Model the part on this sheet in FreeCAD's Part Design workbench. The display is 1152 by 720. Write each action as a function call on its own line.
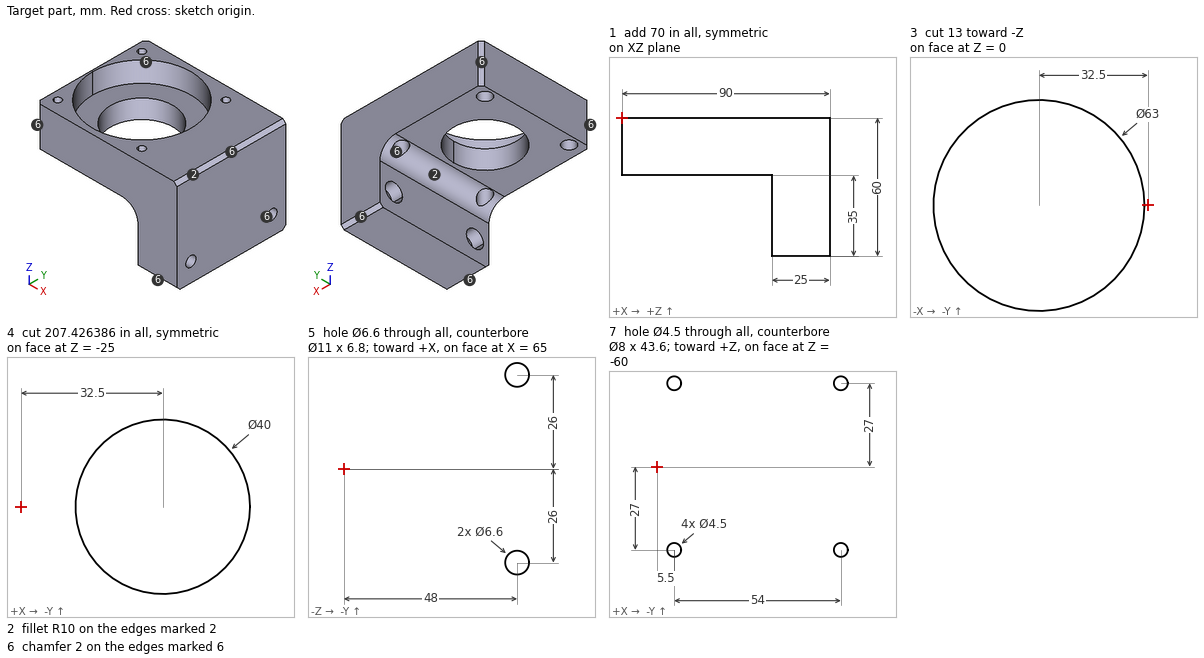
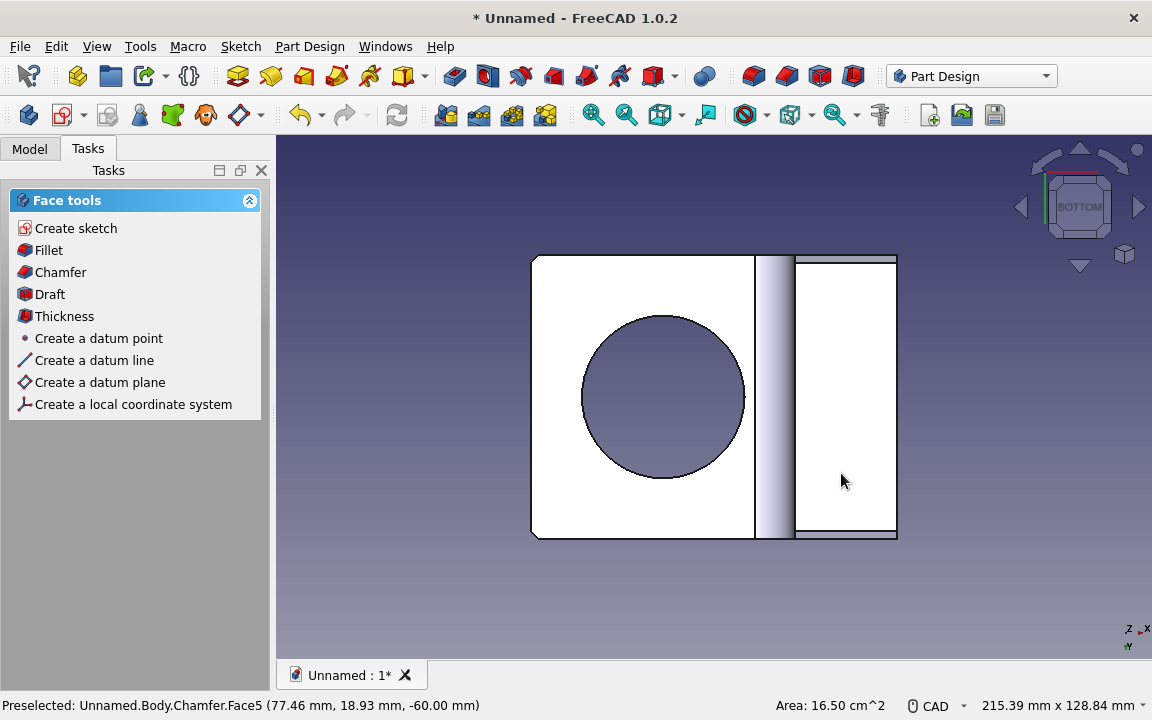
click(62, 116)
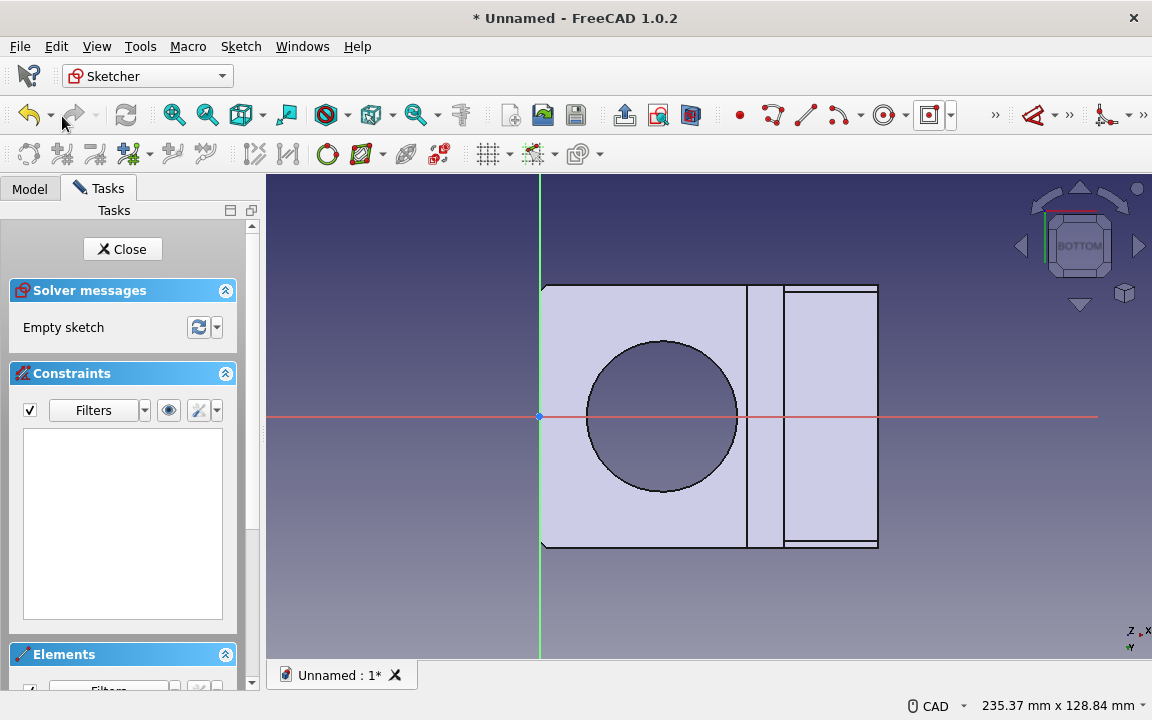
scroll(687, 417, up, 2)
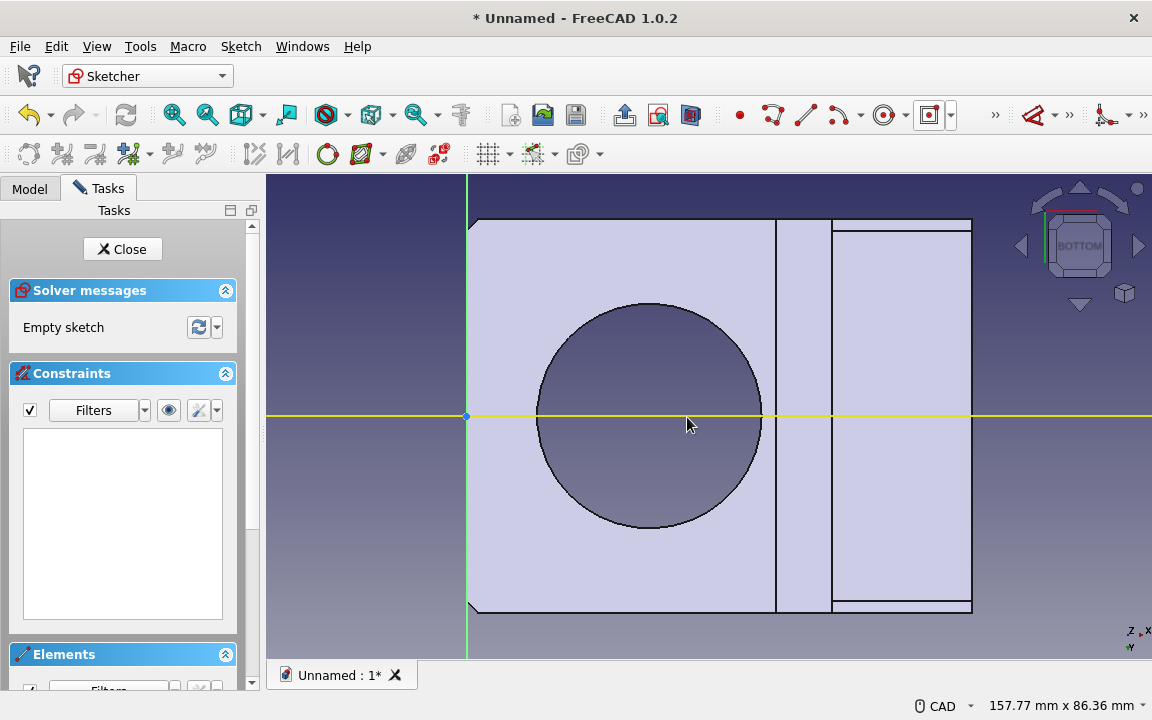
click(884, 116)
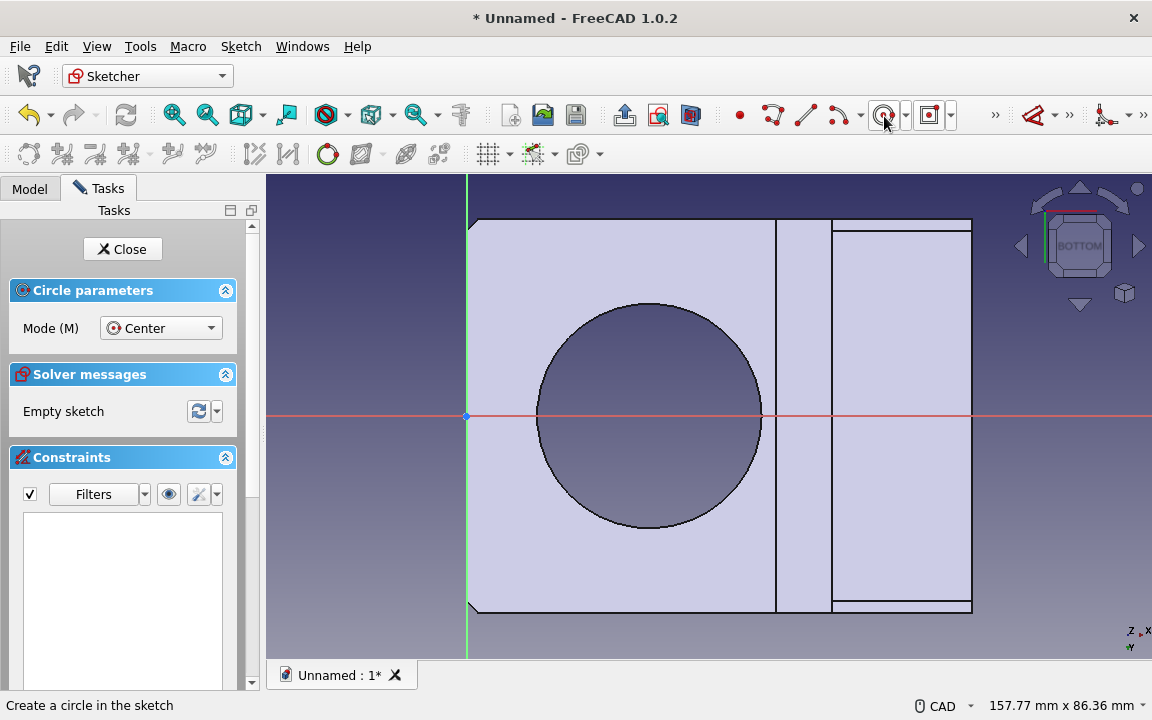
scroll(498, 568, up, 3)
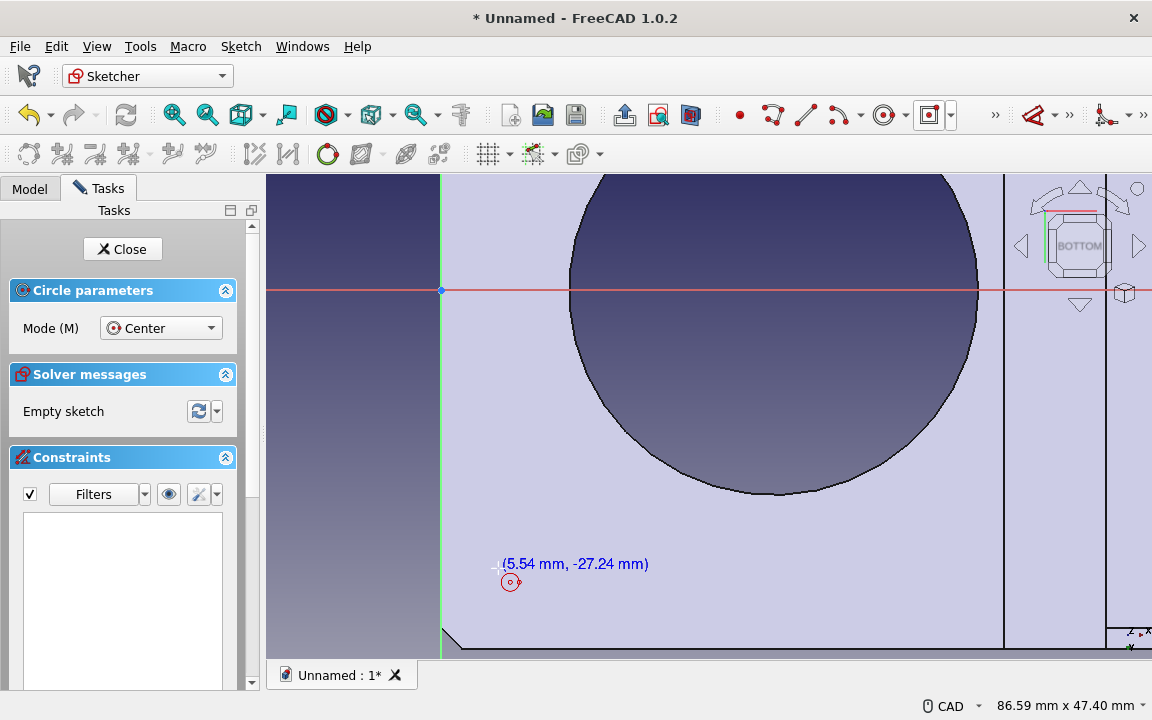
click(497, 567)
move(514, 550)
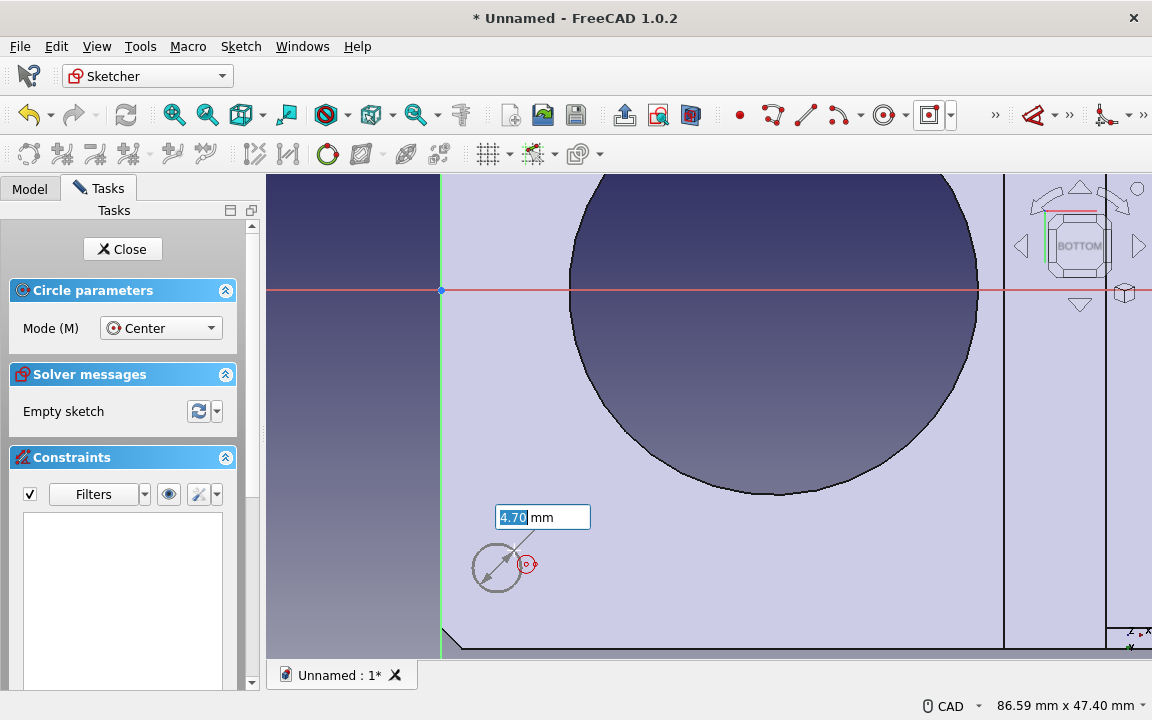
text(4.5)
key(Return)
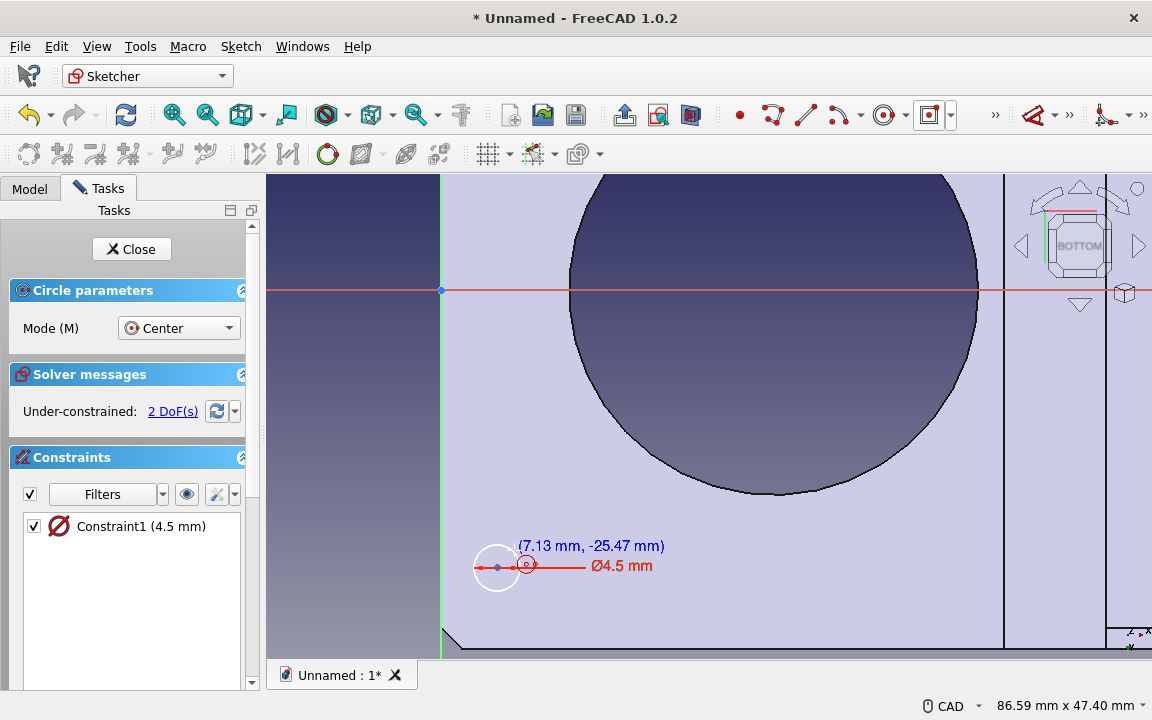
scroll(499, 570, down, 3)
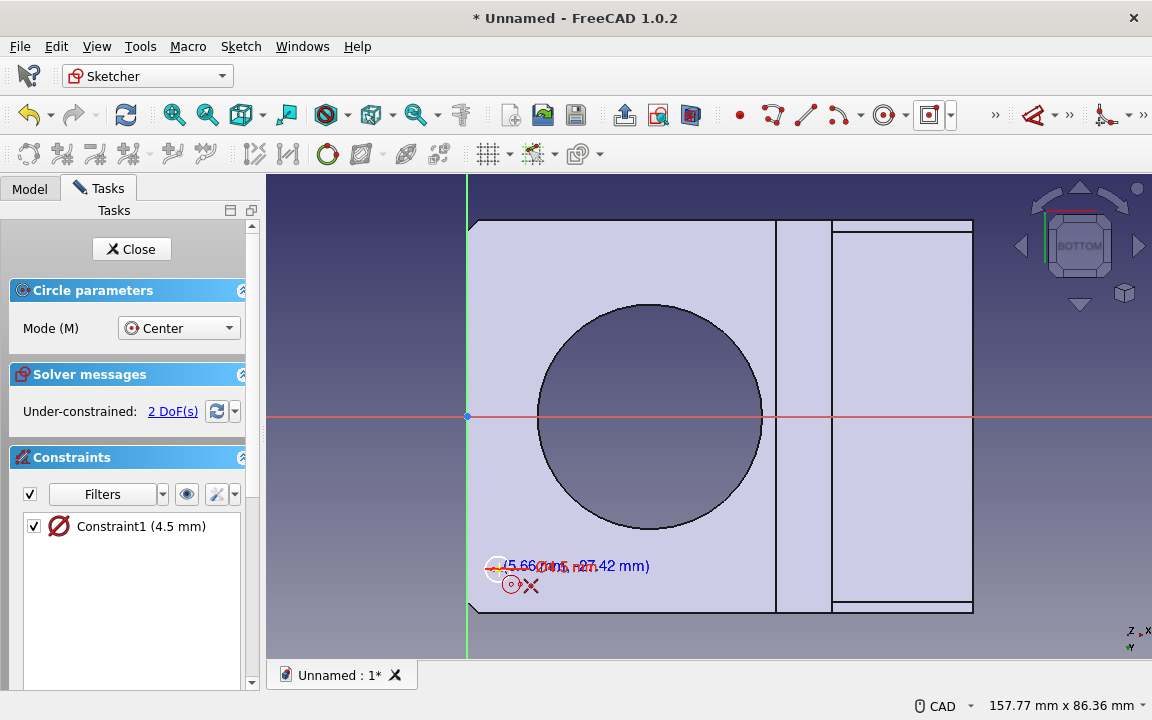
scroll(801, 569, up, 3)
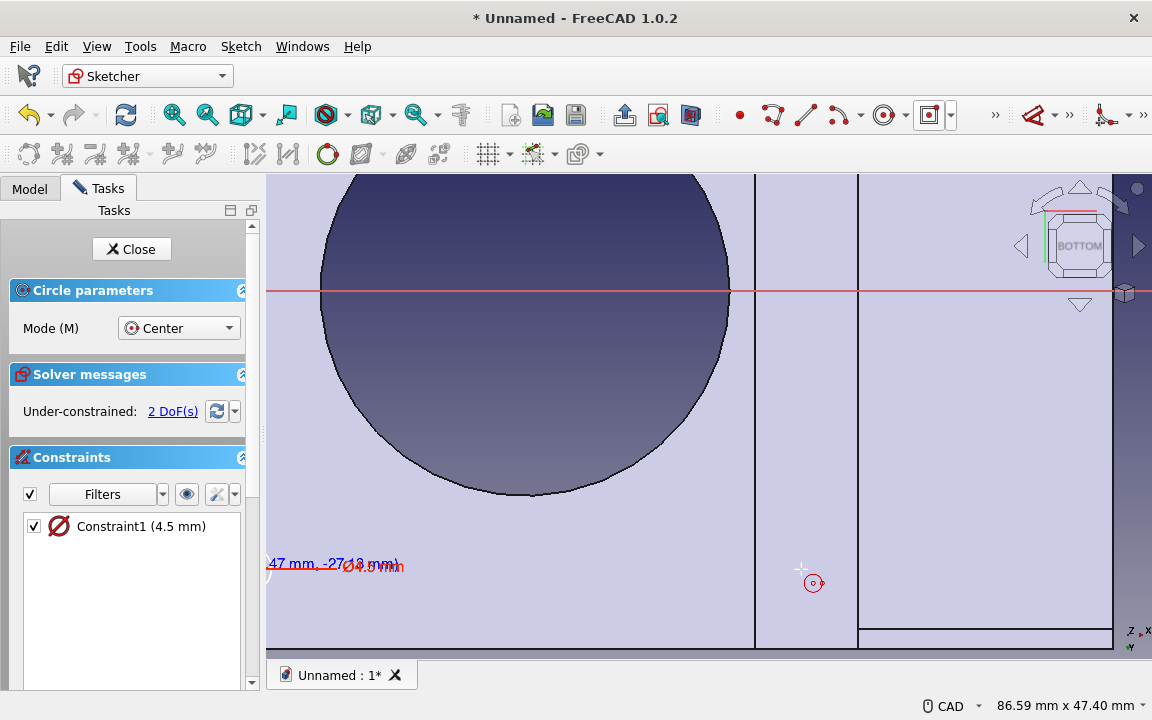
click(801, 567)
move(818, 551)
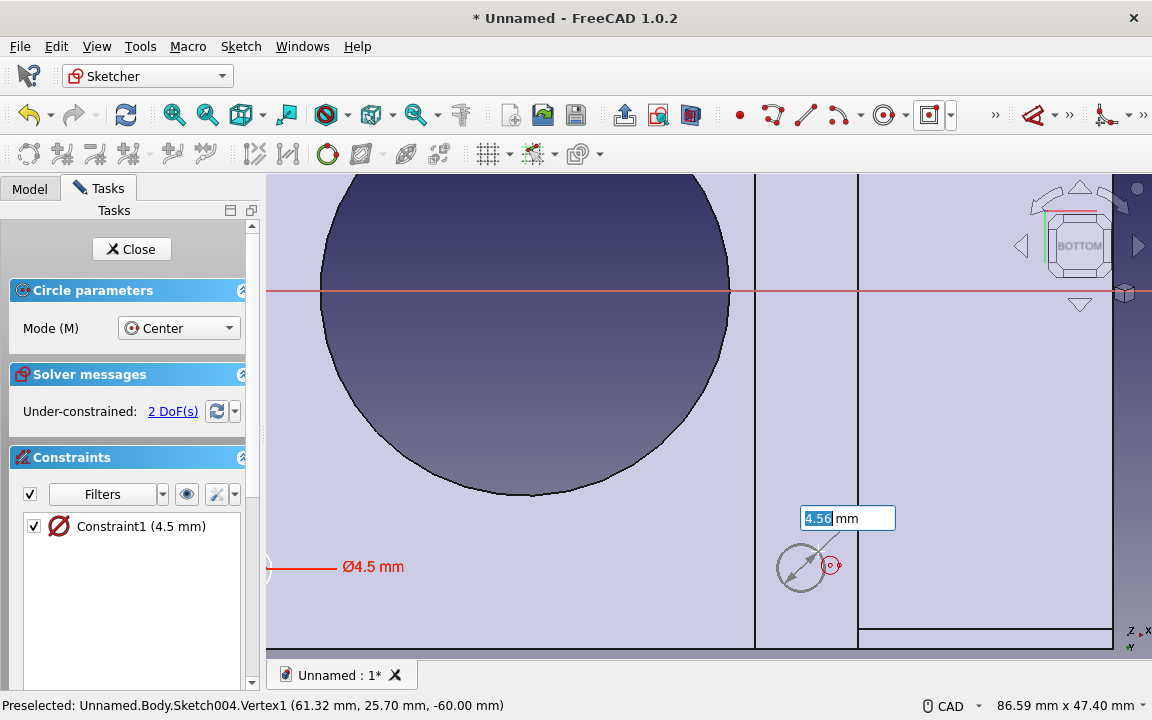
text(4.5)
key(Return)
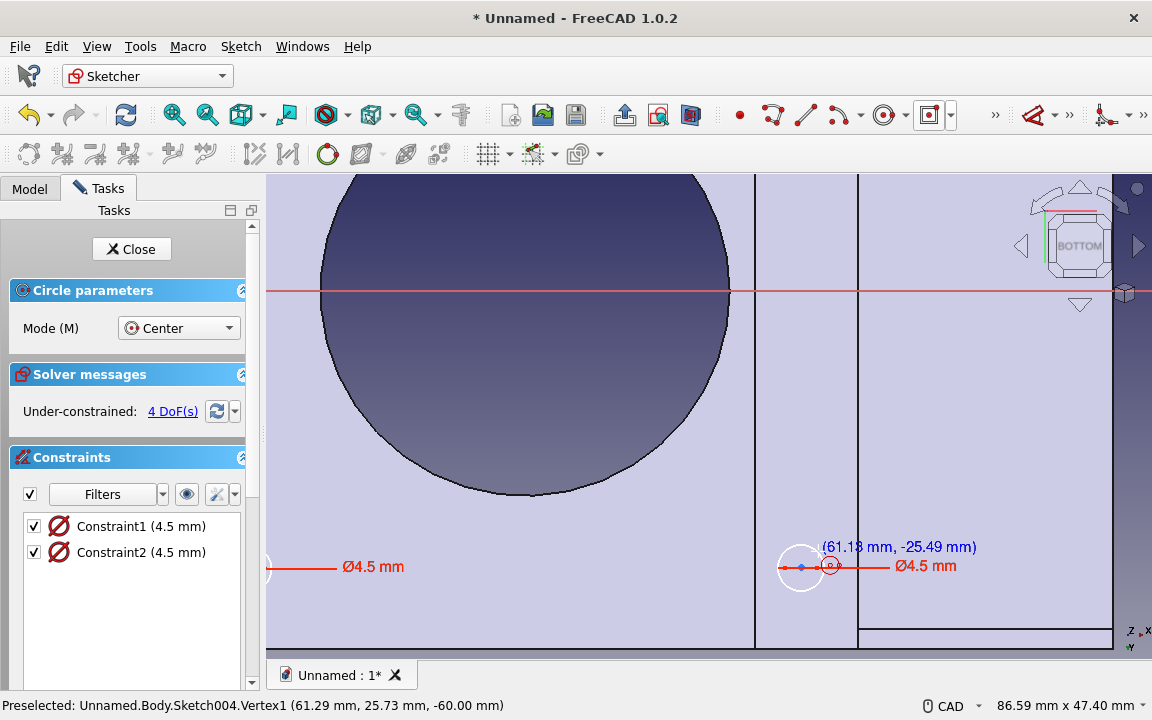
scroll(801, 569, down, 3)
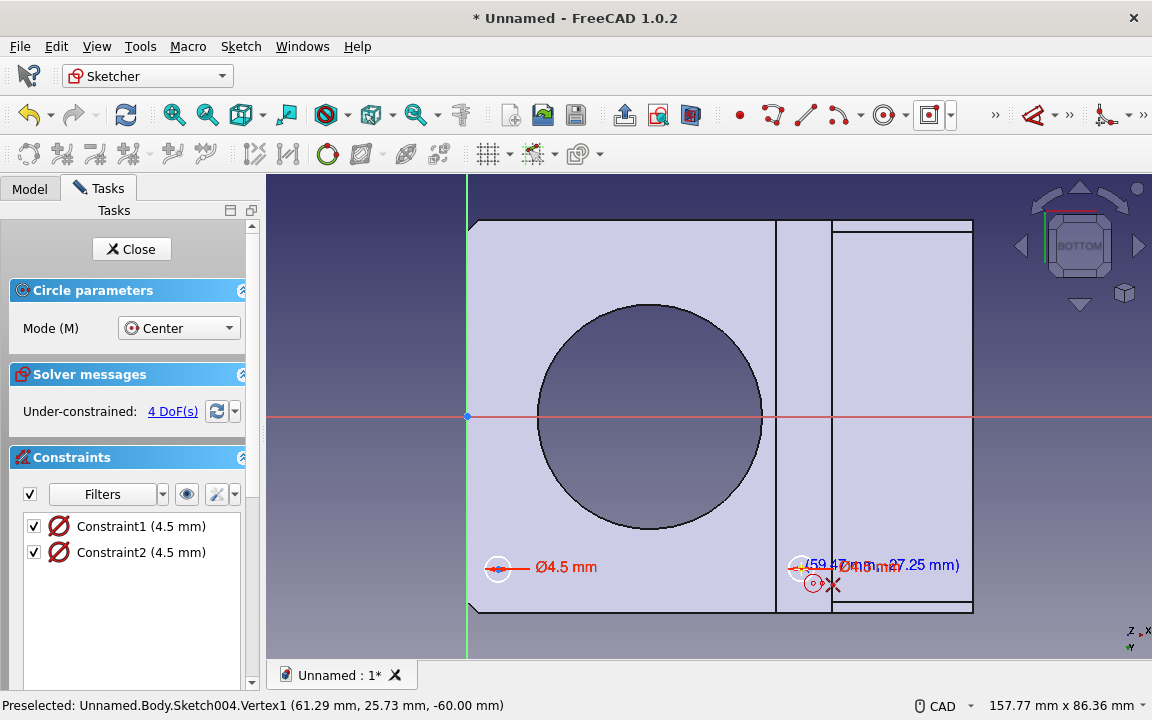
scroll(801, 265, up, 3)